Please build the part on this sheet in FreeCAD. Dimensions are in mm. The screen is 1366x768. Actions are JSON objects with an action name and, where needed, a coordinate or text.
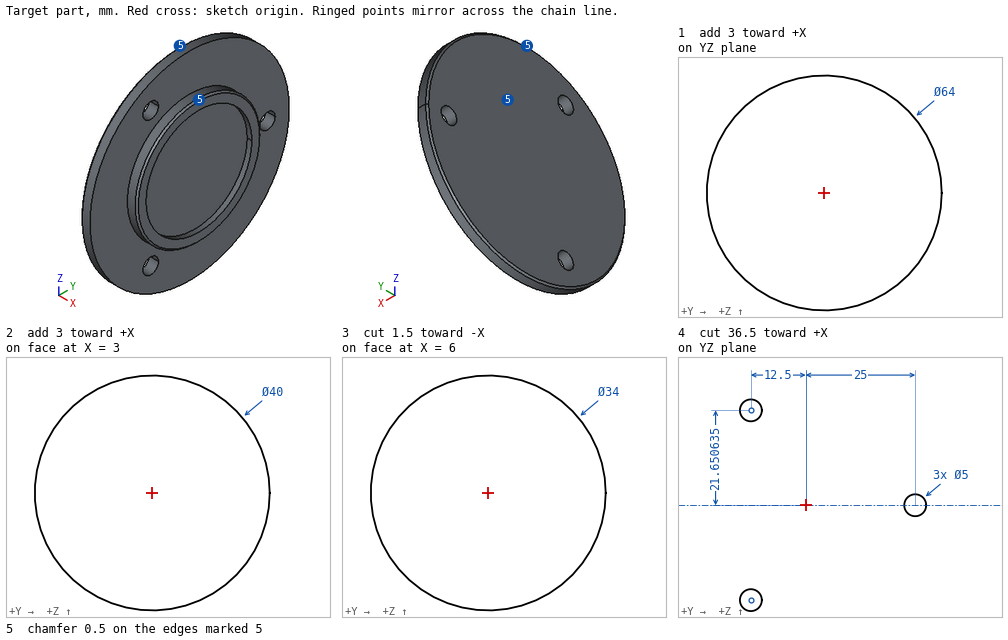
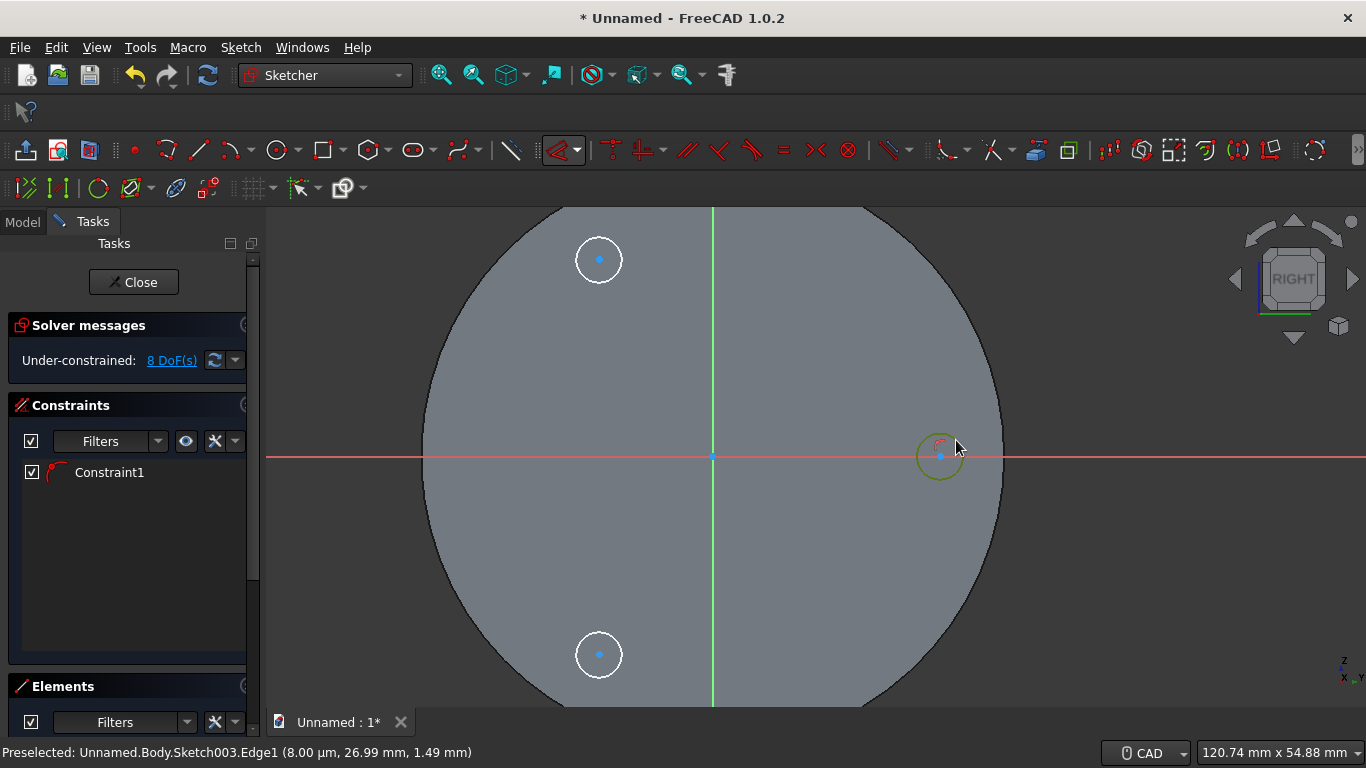
{"action": "left_click", "coordinate": [615, 244]}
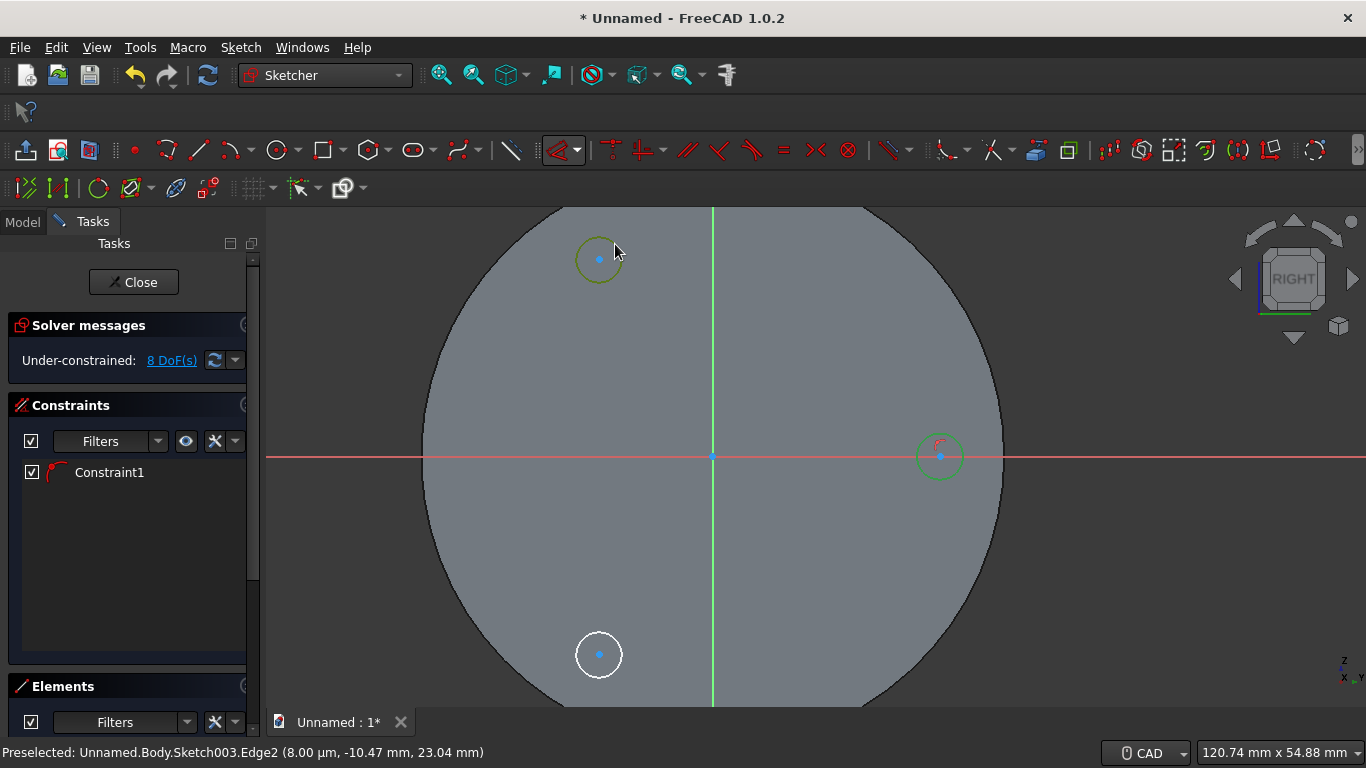
{"action": "left_click", "coordinate": [615, 639]}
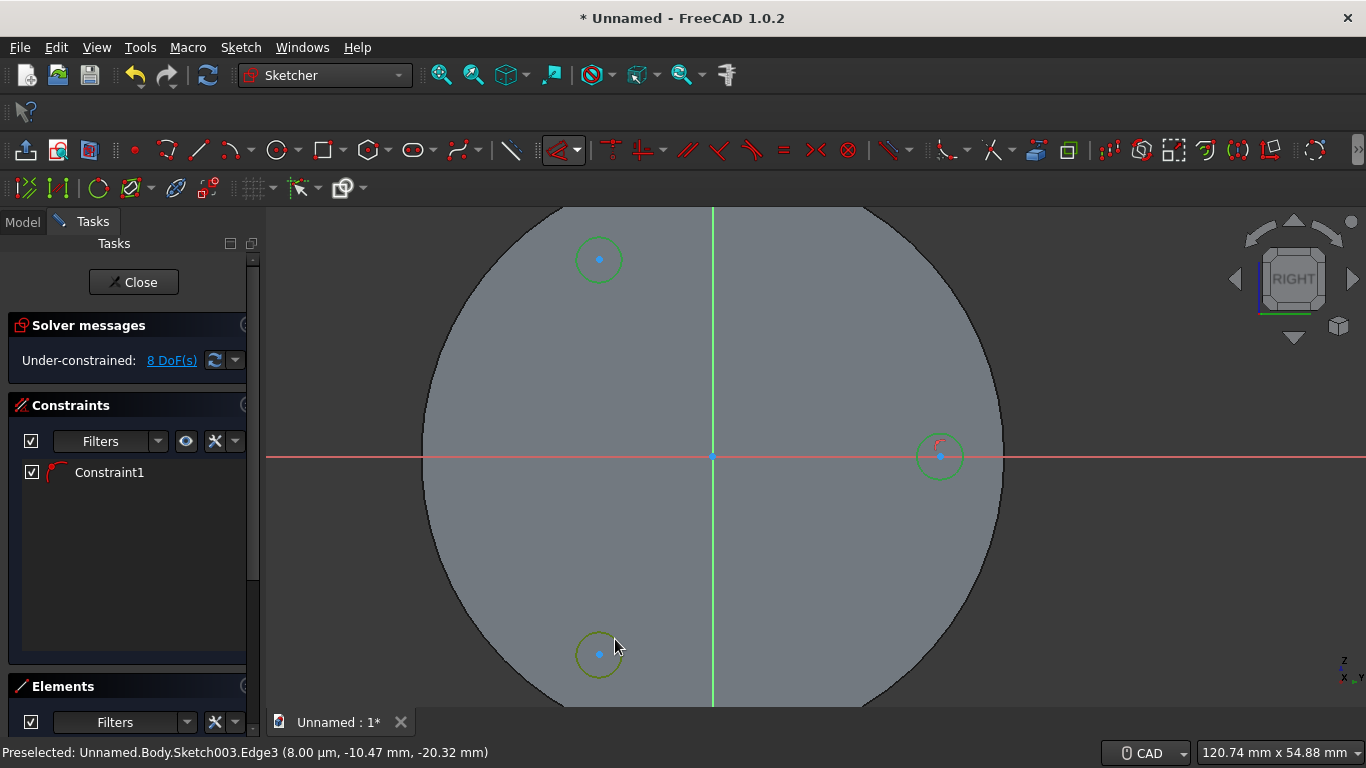
{"action": "left_click", "coordinate": [784, 150]}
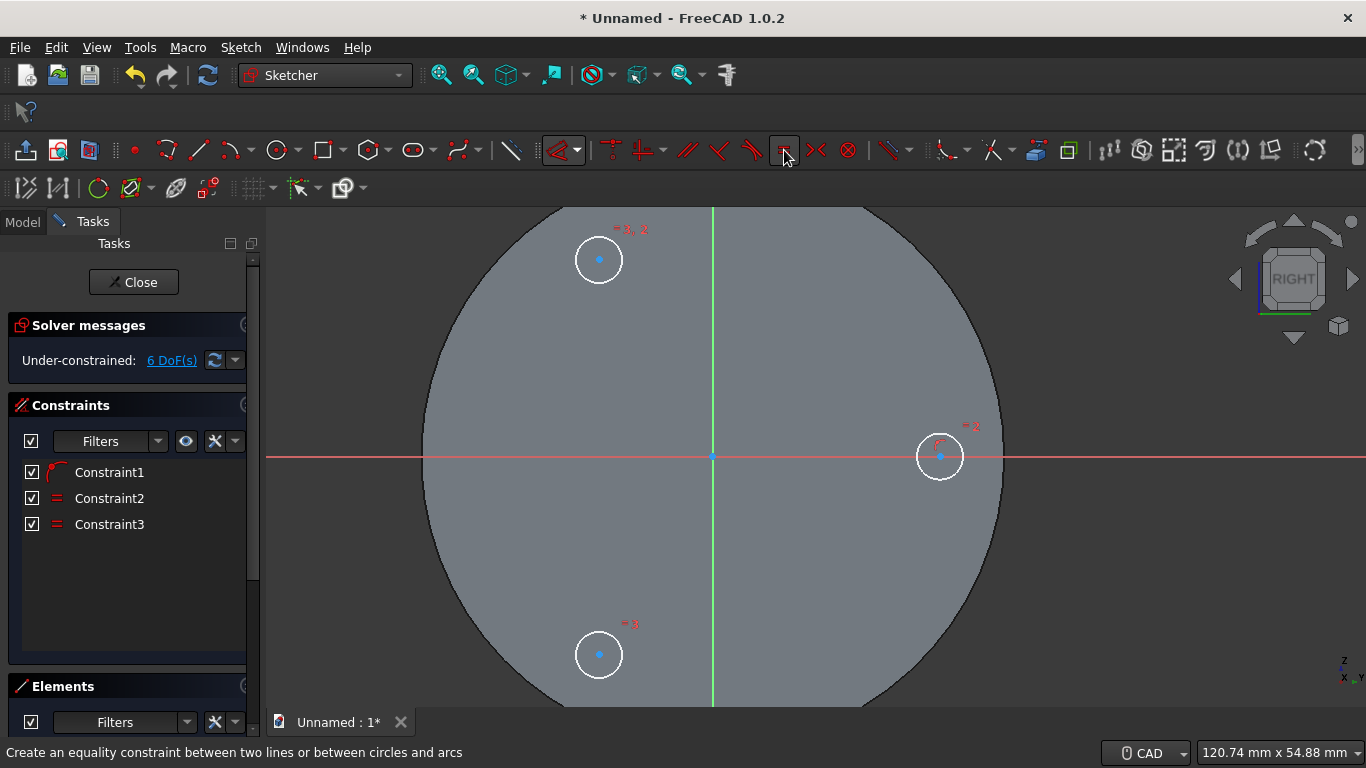
{"action": "left_click", "coordinate": [599, 260]}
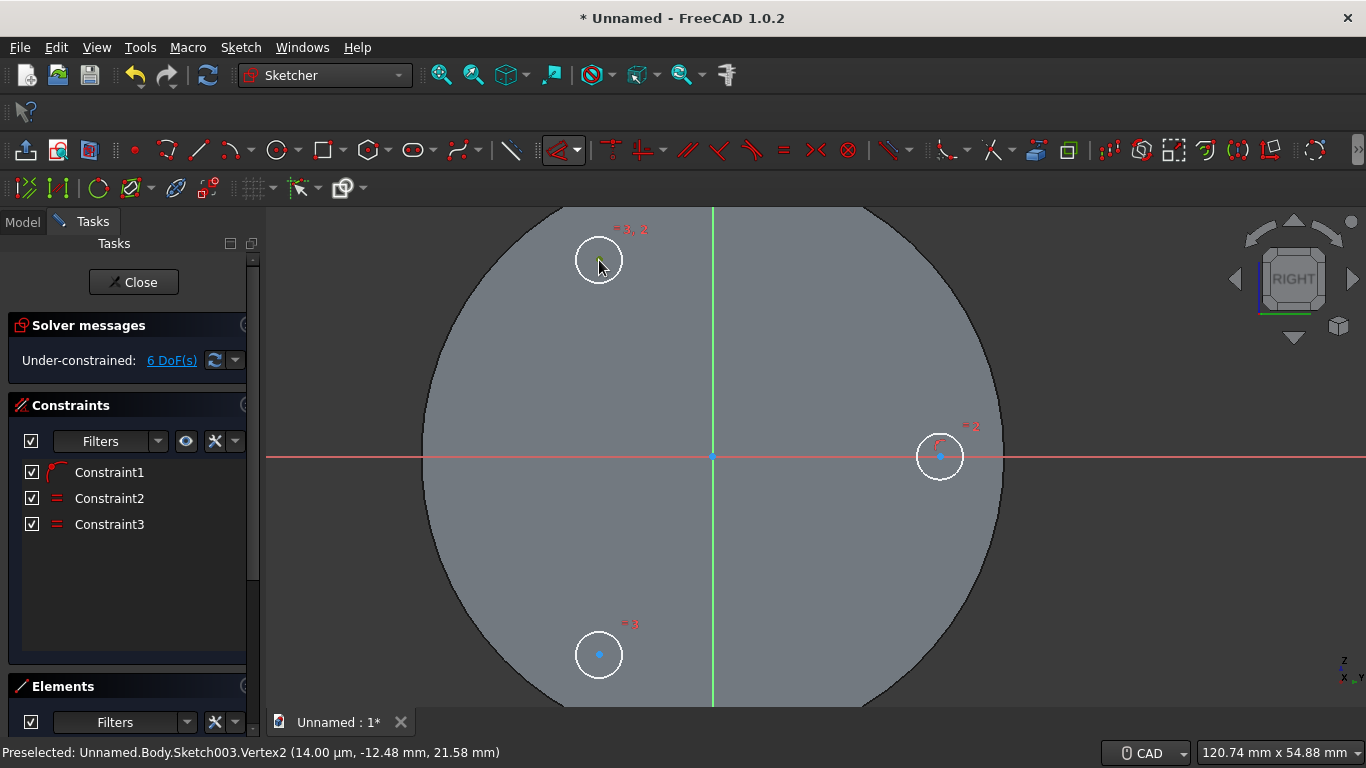
{"action": "left_click", "coordinate": [599, 655]}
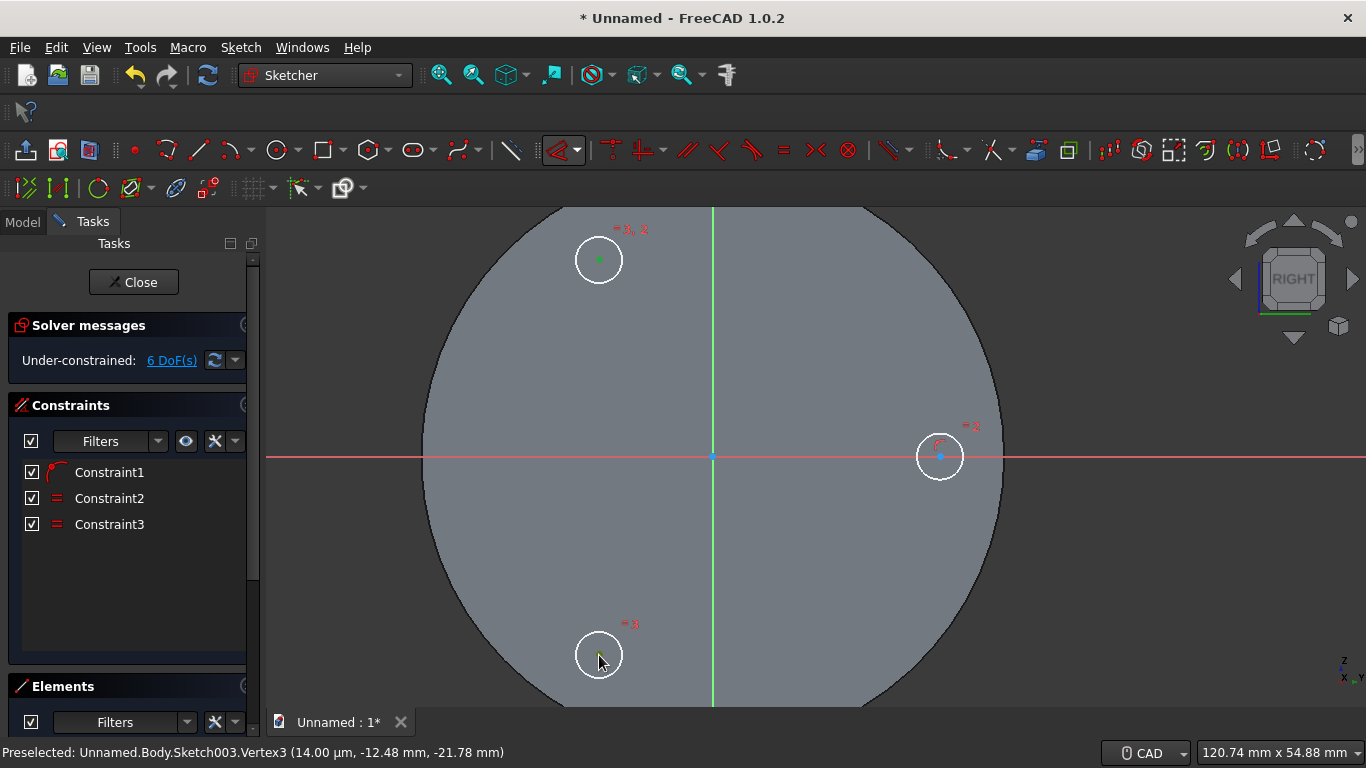
{"action": "left_click", "coordinate": [359, 457]}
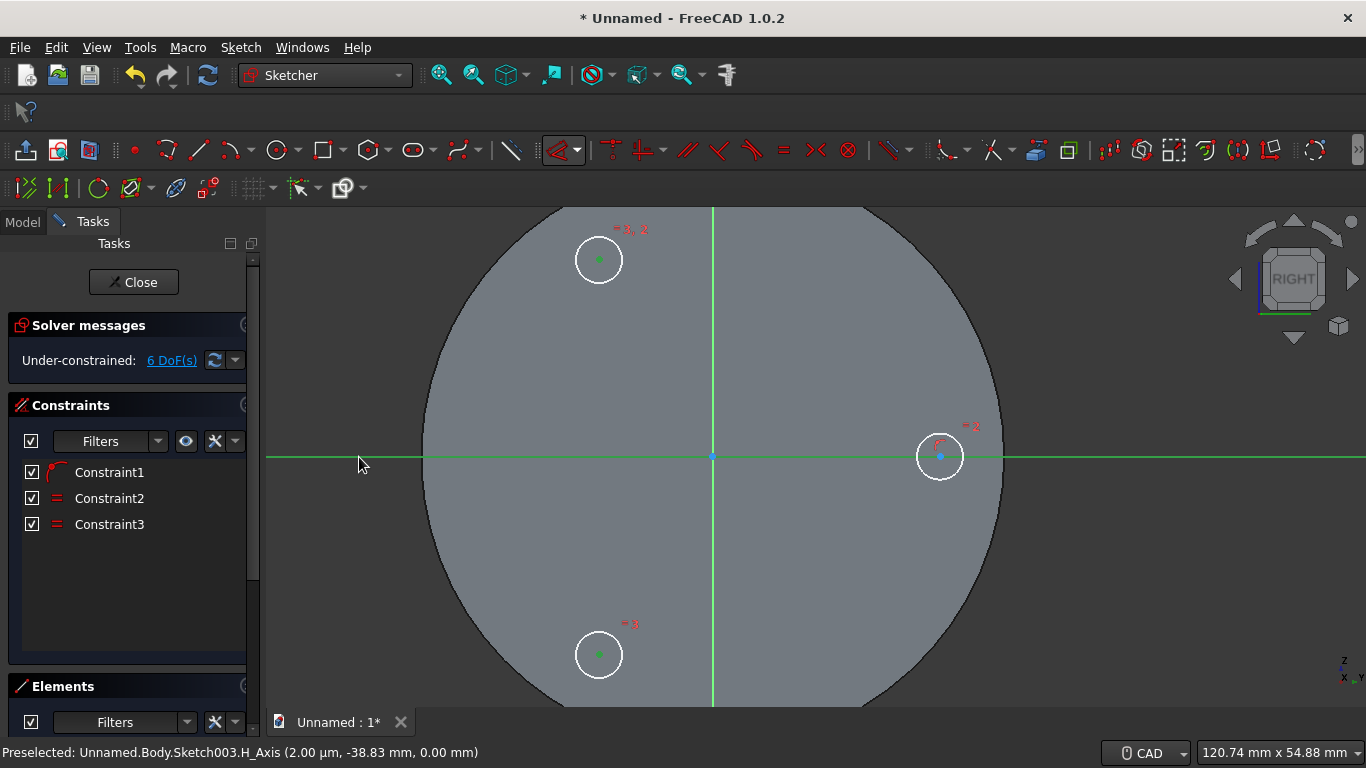
{"action": "left_click", "coordinate": [816, 150]}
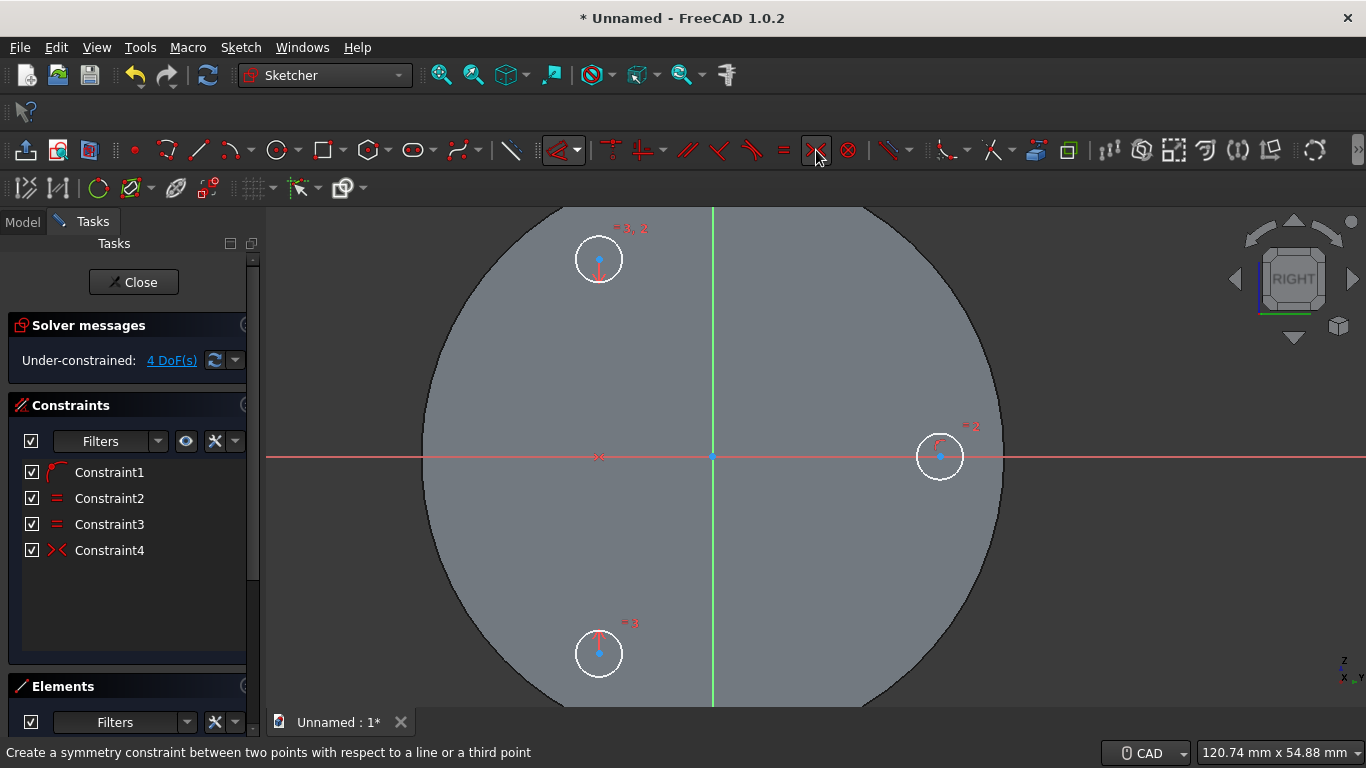
{"action": "left_click", "coordinate": [956, 440]}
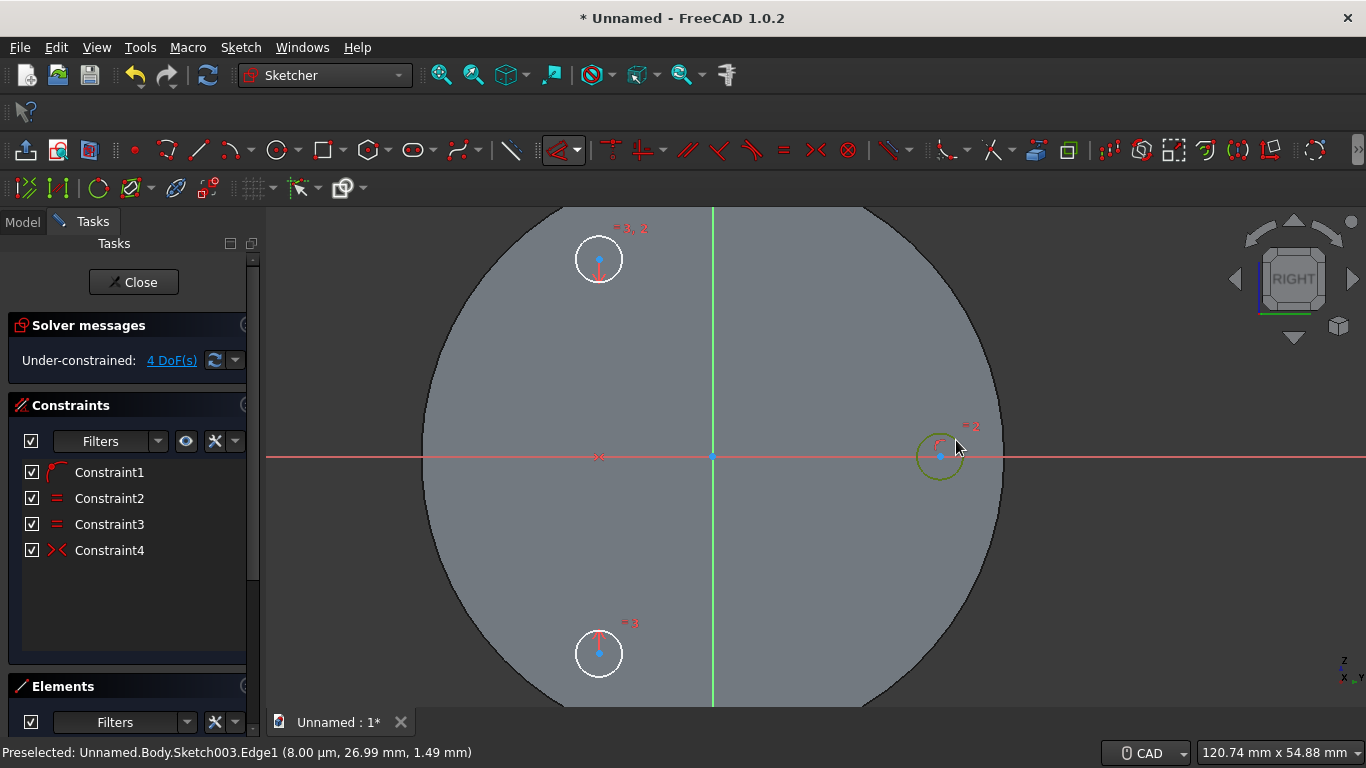
{"action": "key", "text": "k o"}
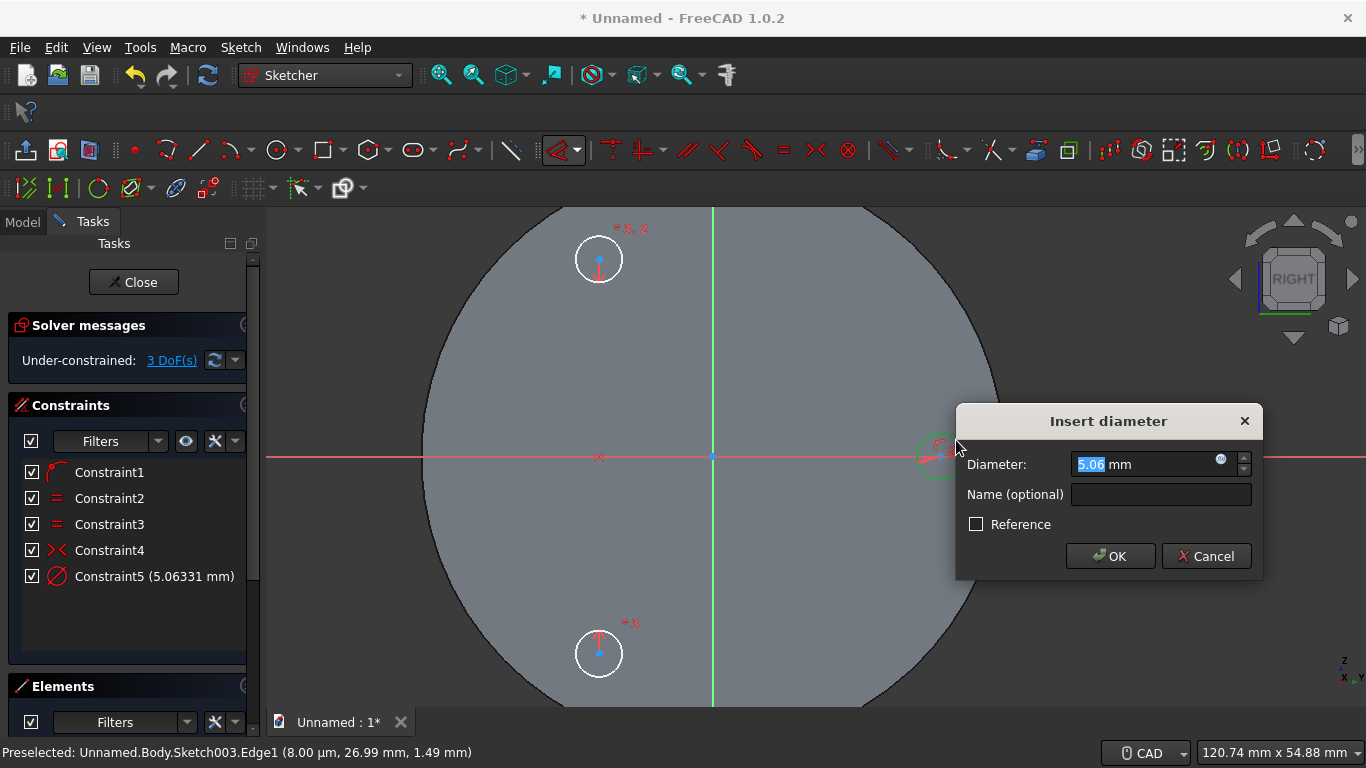
{"action": "type", "text": "5"}
{"action": "key", "text": "Return"}